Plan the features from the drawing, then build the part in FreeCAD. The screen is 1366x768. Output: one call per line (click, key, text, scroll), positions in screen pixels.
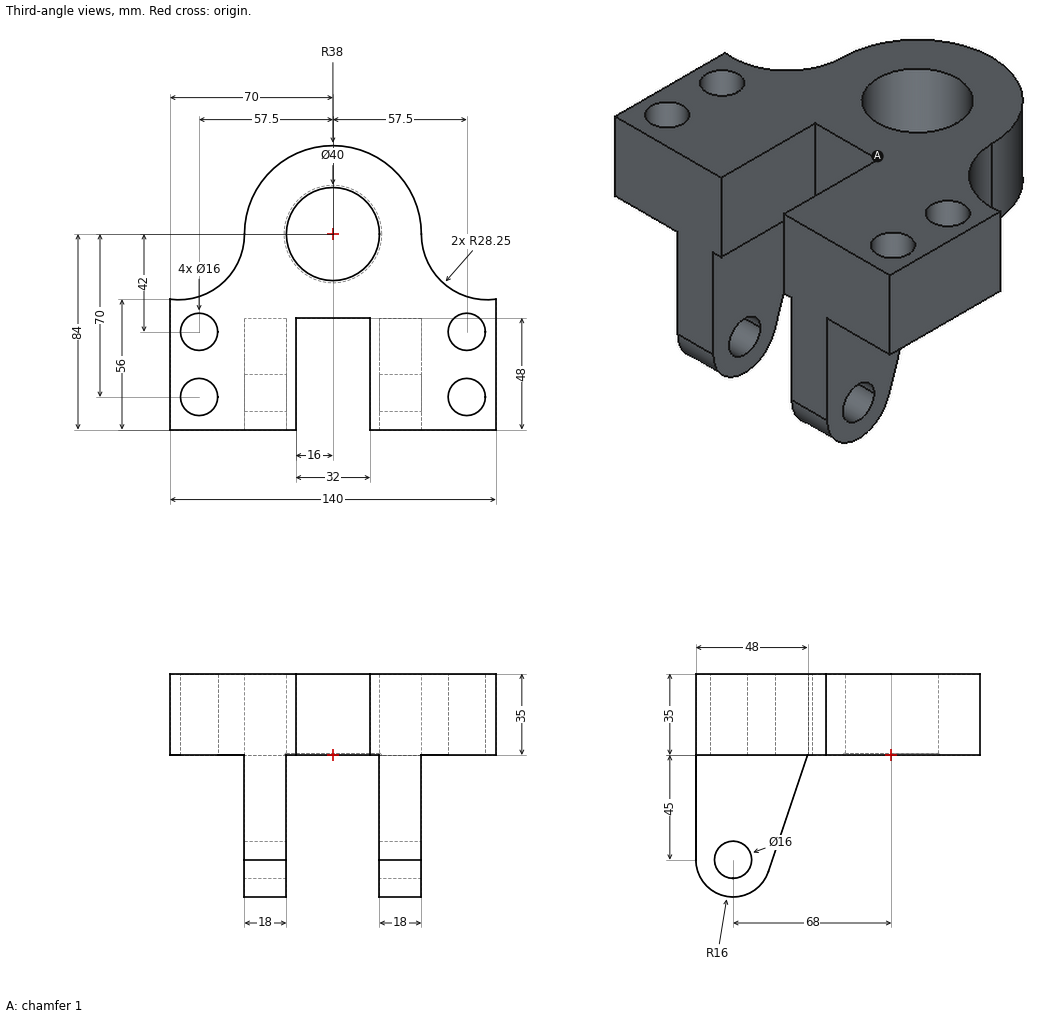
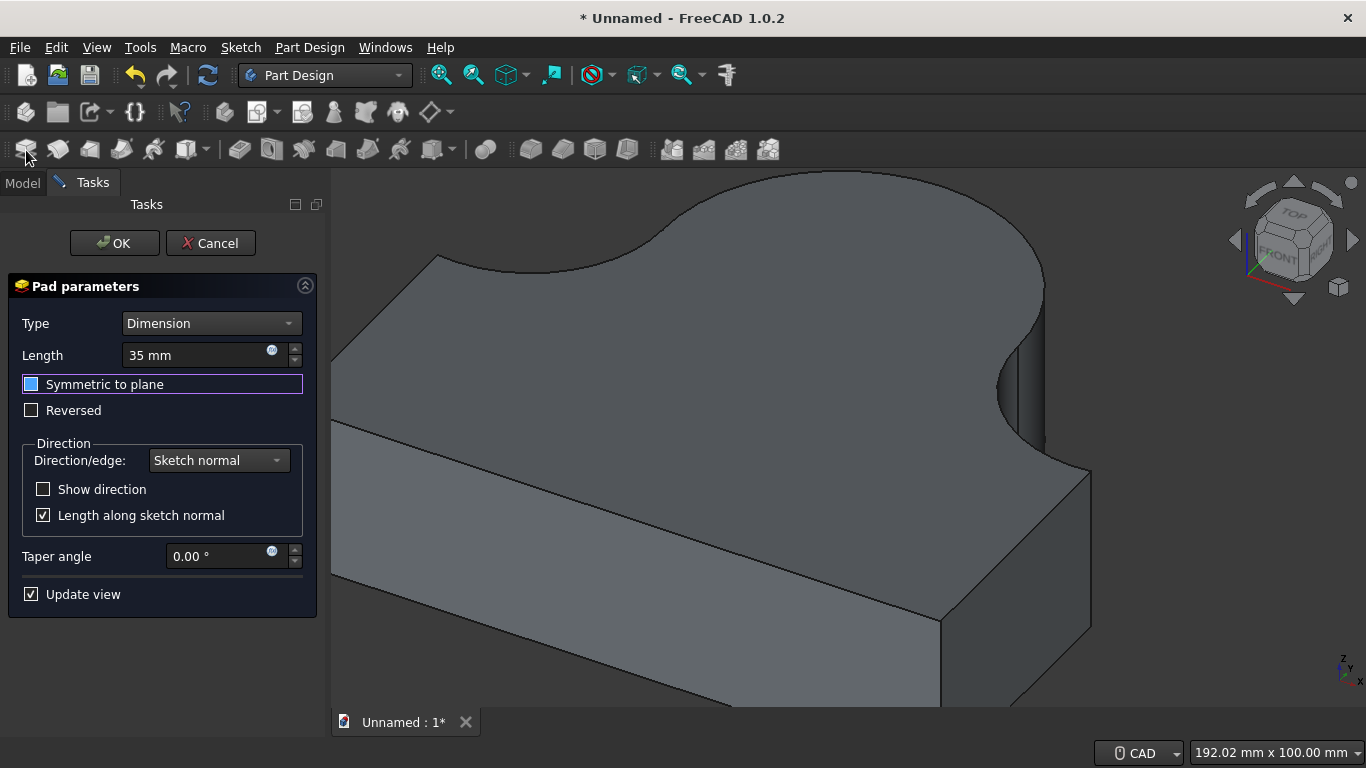
click(115, 243)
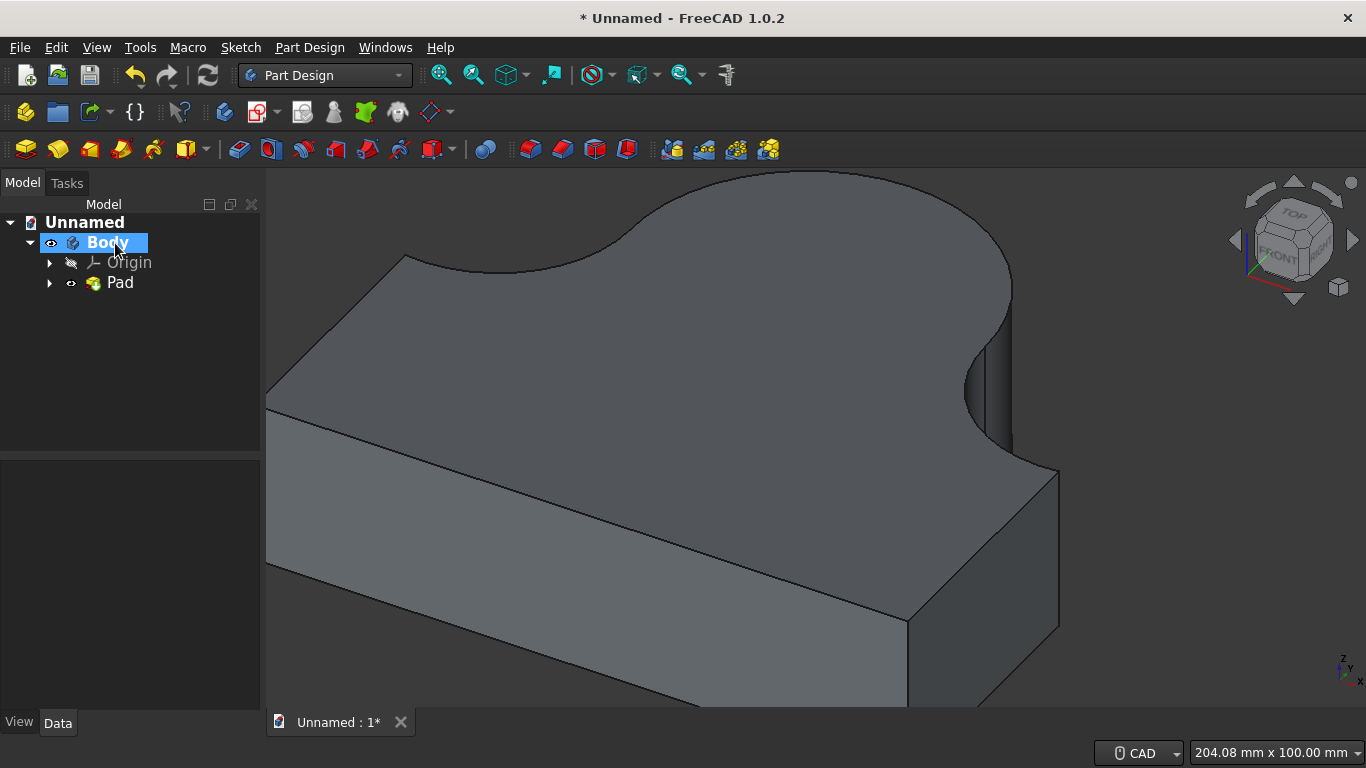
key(v)
key(f)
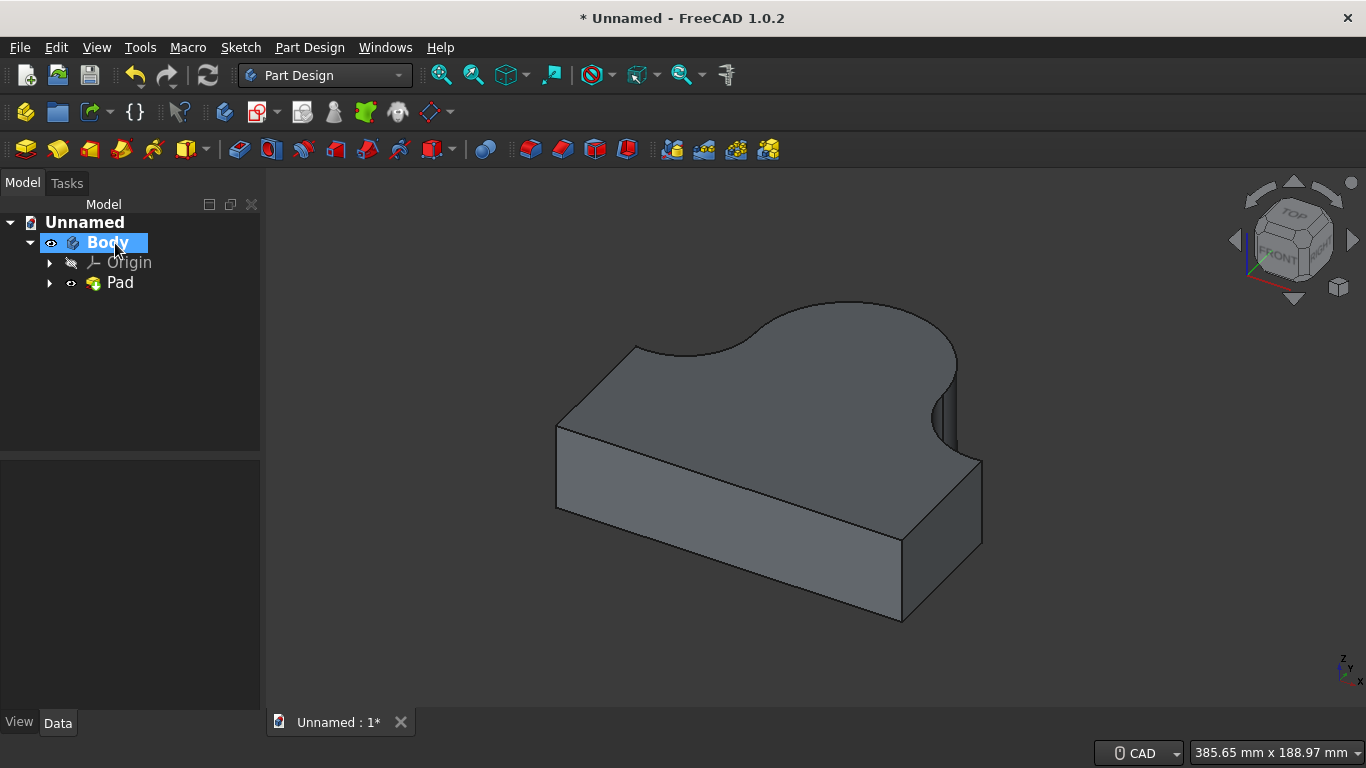
click(791, 420)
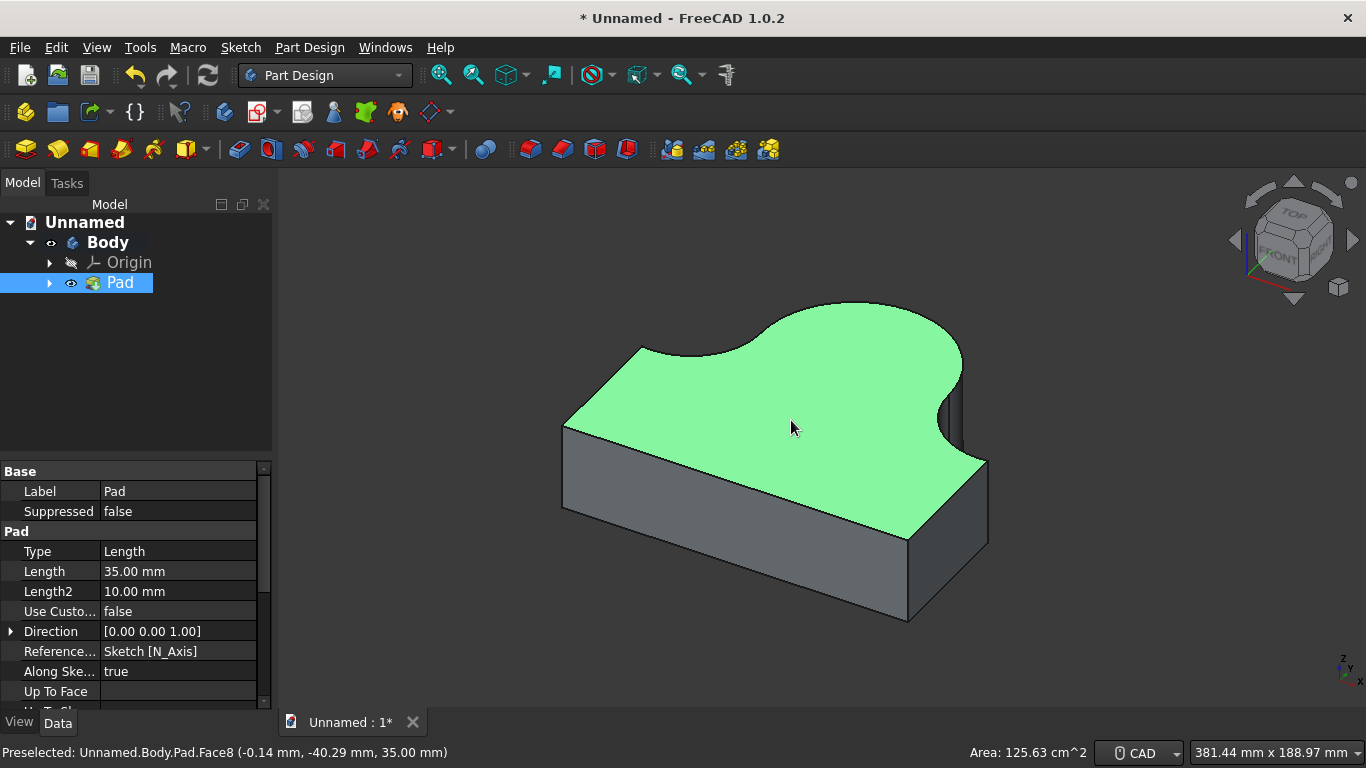
click(258, 112)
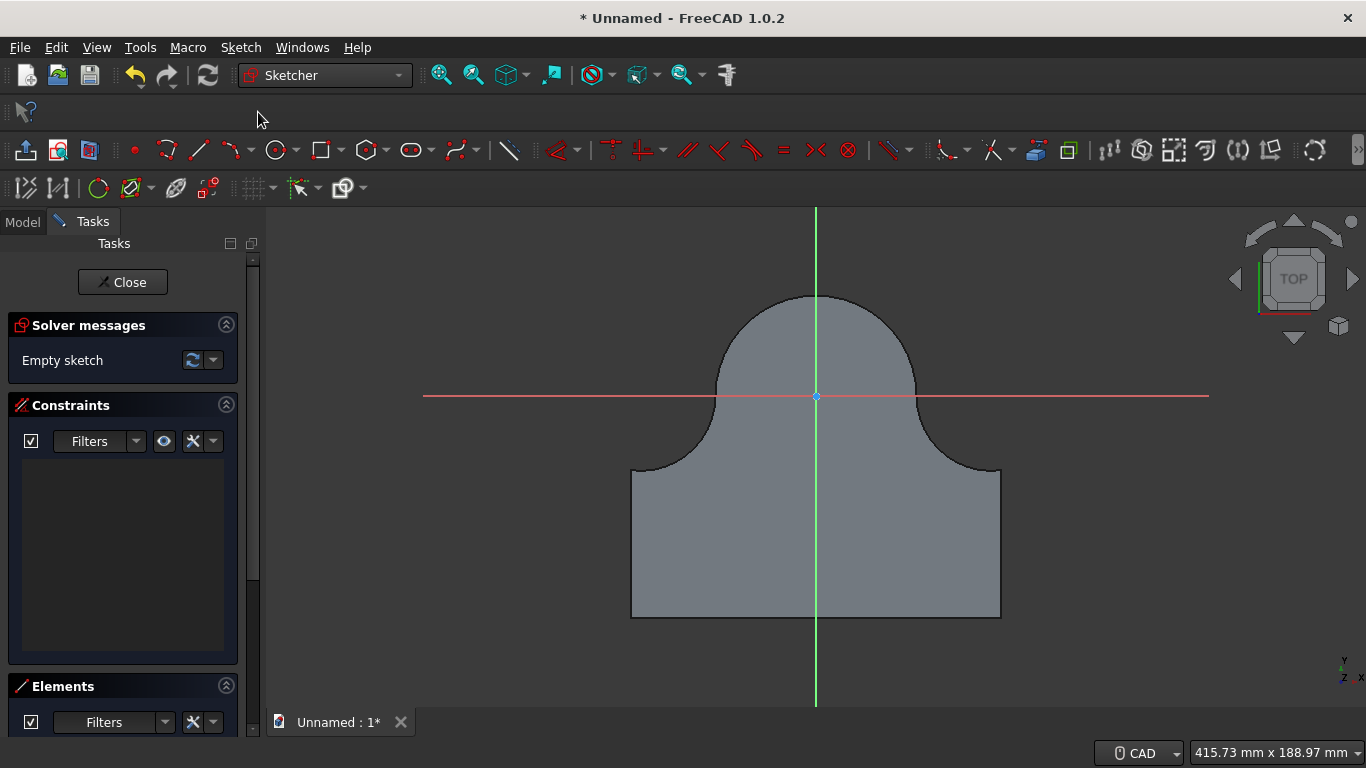
scroll(856, 361, up, 5)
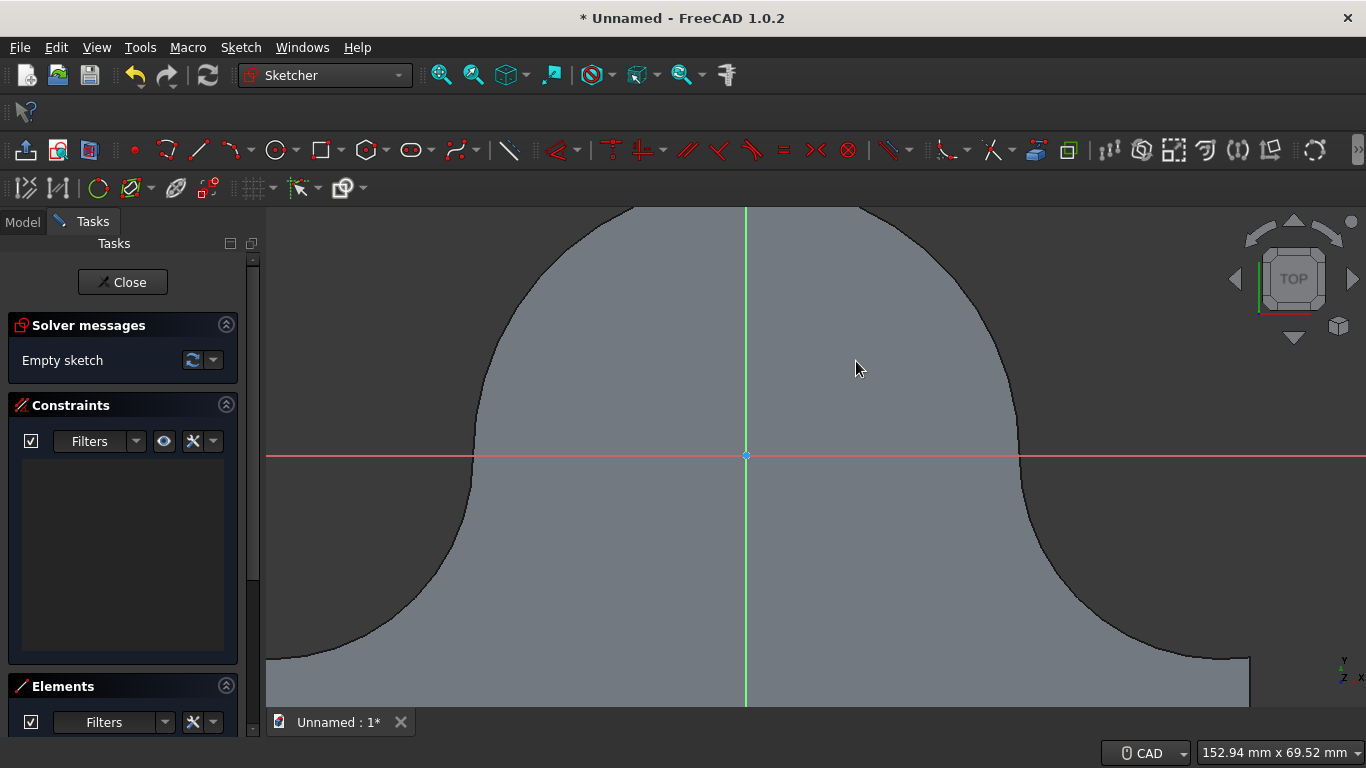
key(g)
key(c)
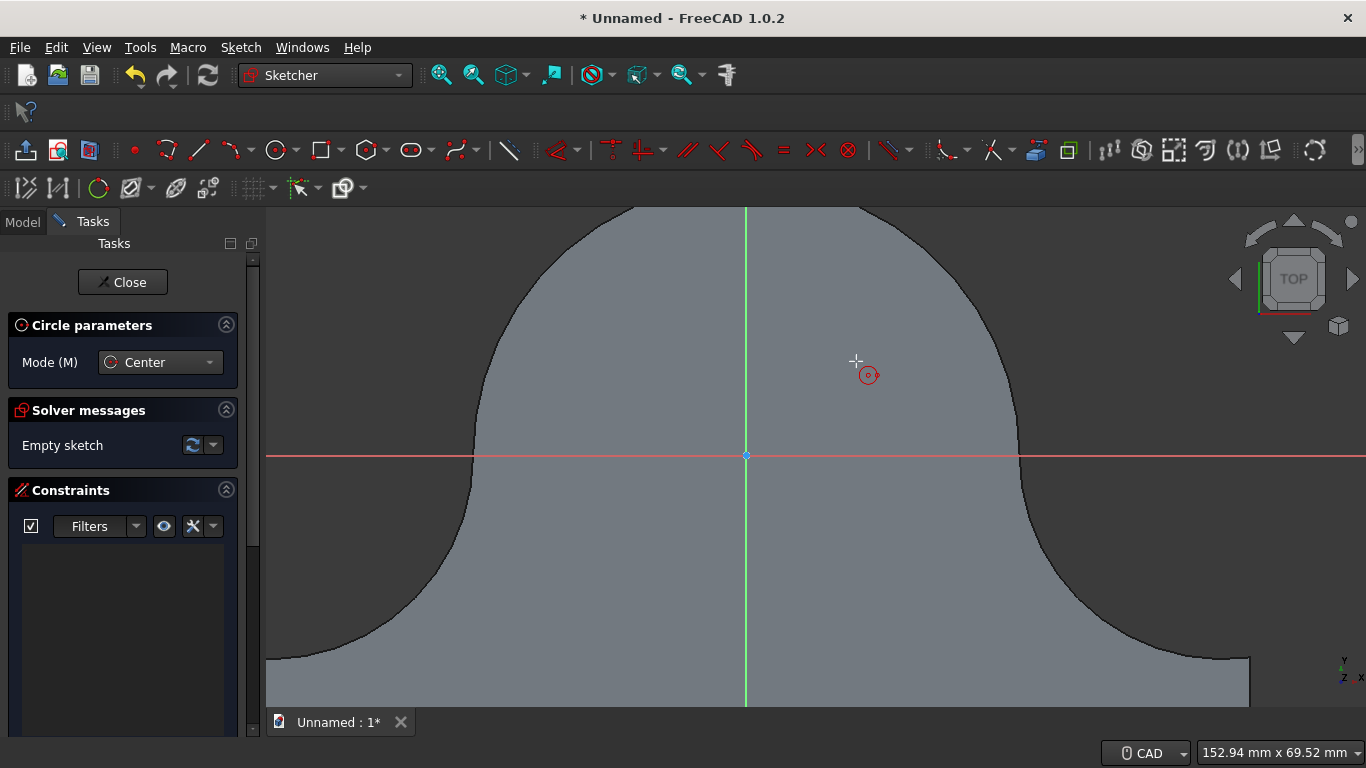
click(746, 456)
move(848, 354)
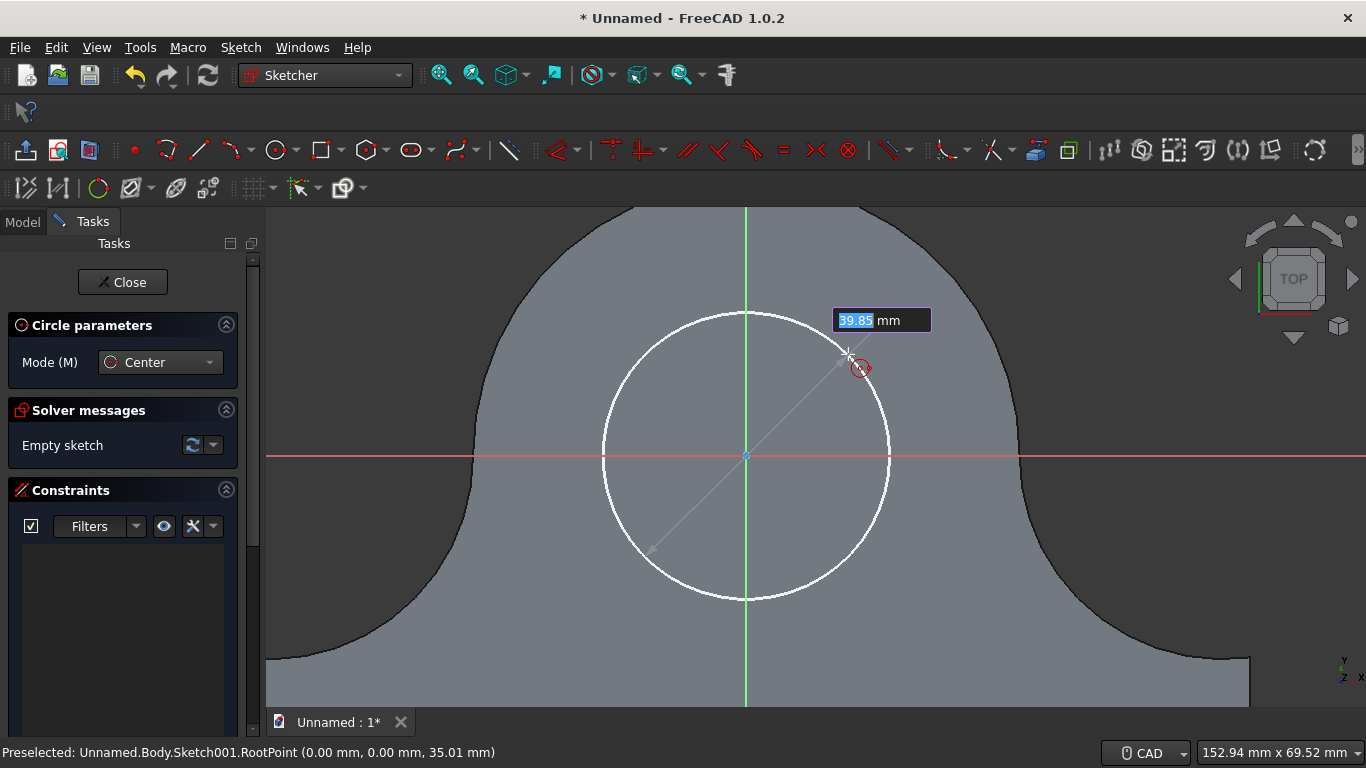
text(40)
key(Return)
key(Escape)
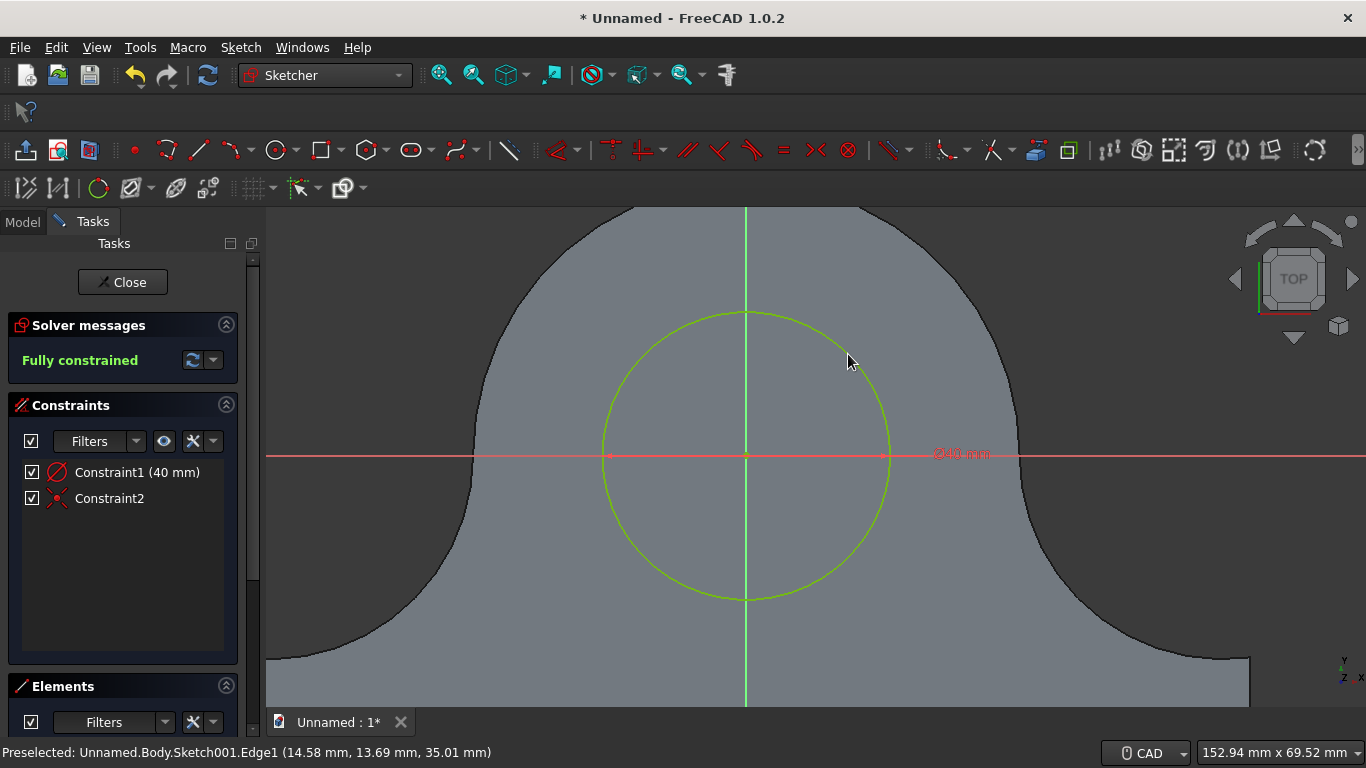
click(123, 282)